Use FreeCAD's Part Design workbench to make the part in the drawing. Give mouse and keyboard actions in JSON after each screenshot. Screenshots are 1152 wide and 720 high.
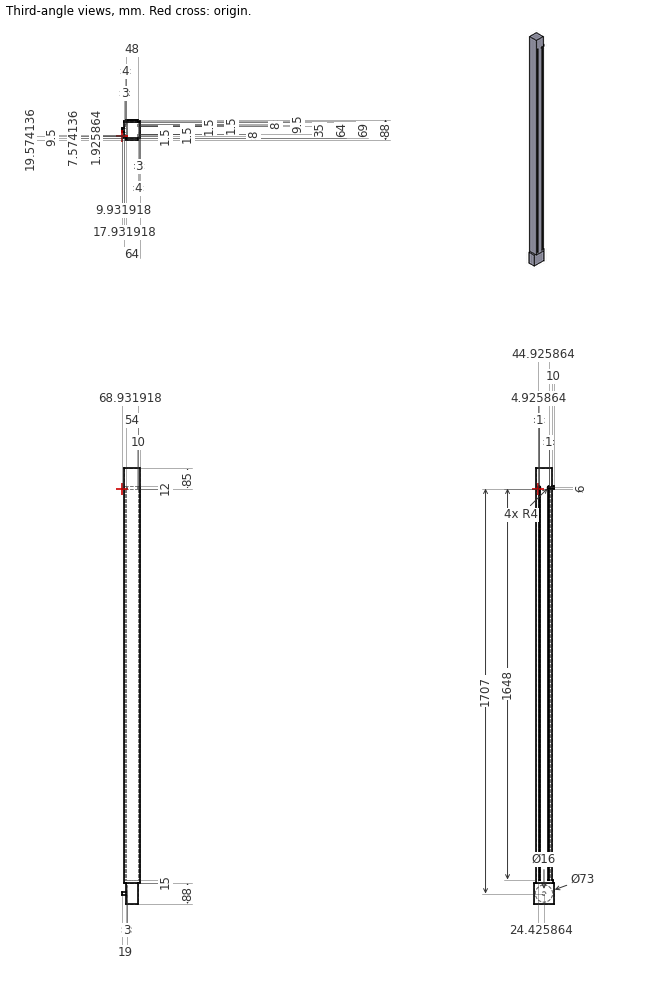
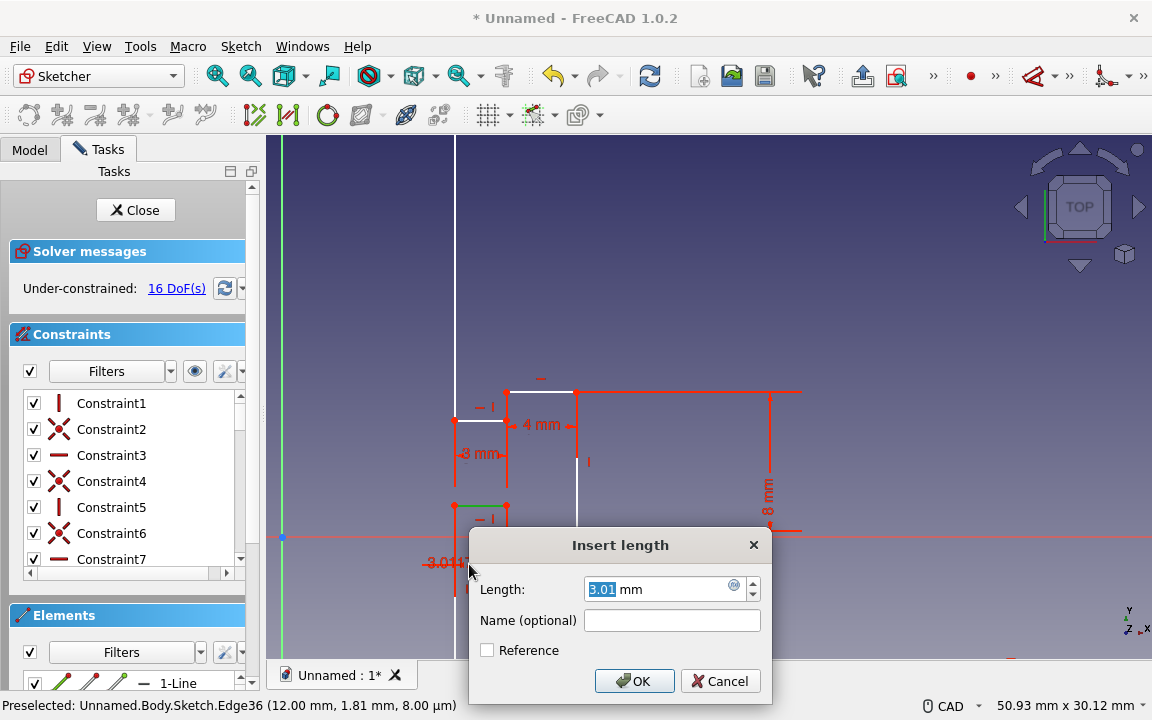
{"action": "type", "text": "3"}
{"action": "key", "text": "Return"}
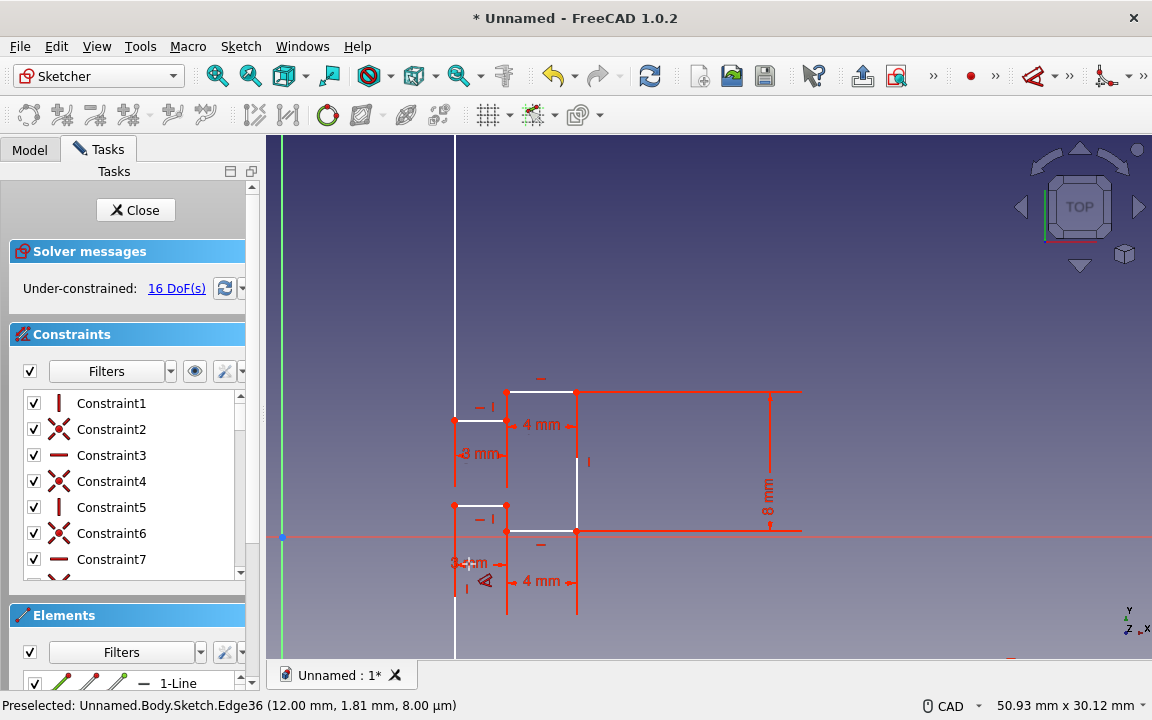
{"action": "scroll", "coordinate": [518, 520], "scroll_direction": "down", "scroll_amount": 6}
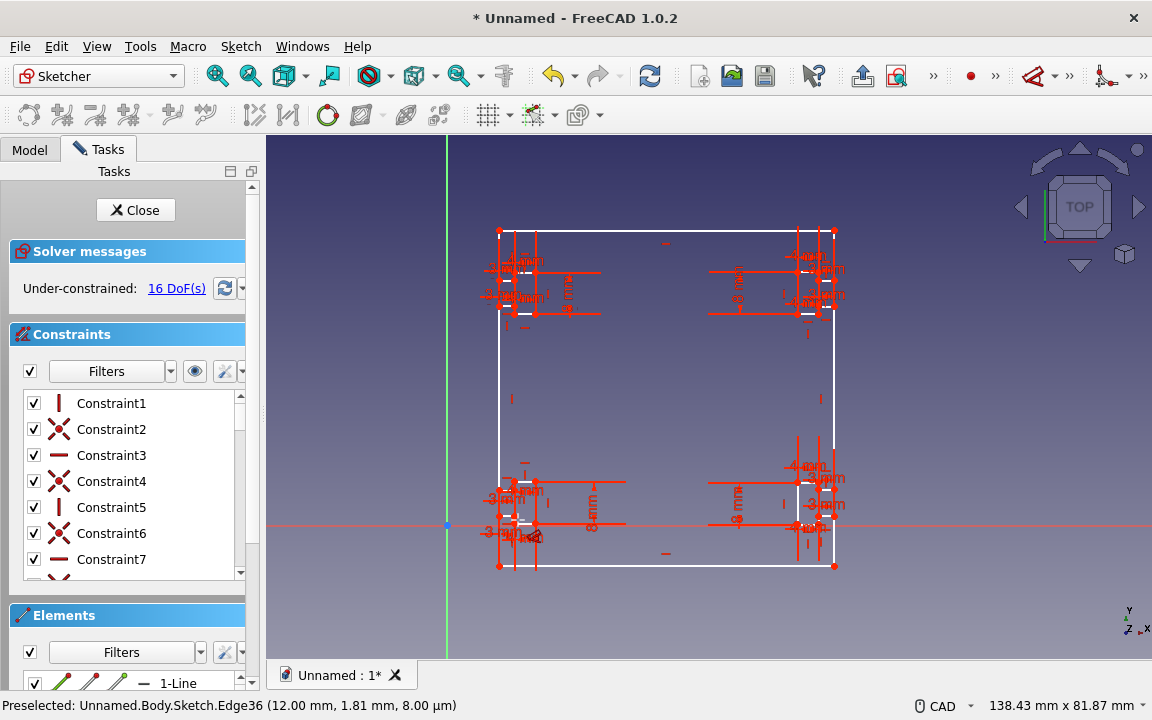
{"action": "left_click", "coordinate": [600, 566]}
{"action": "left_click", "coordinate": [667, 600]}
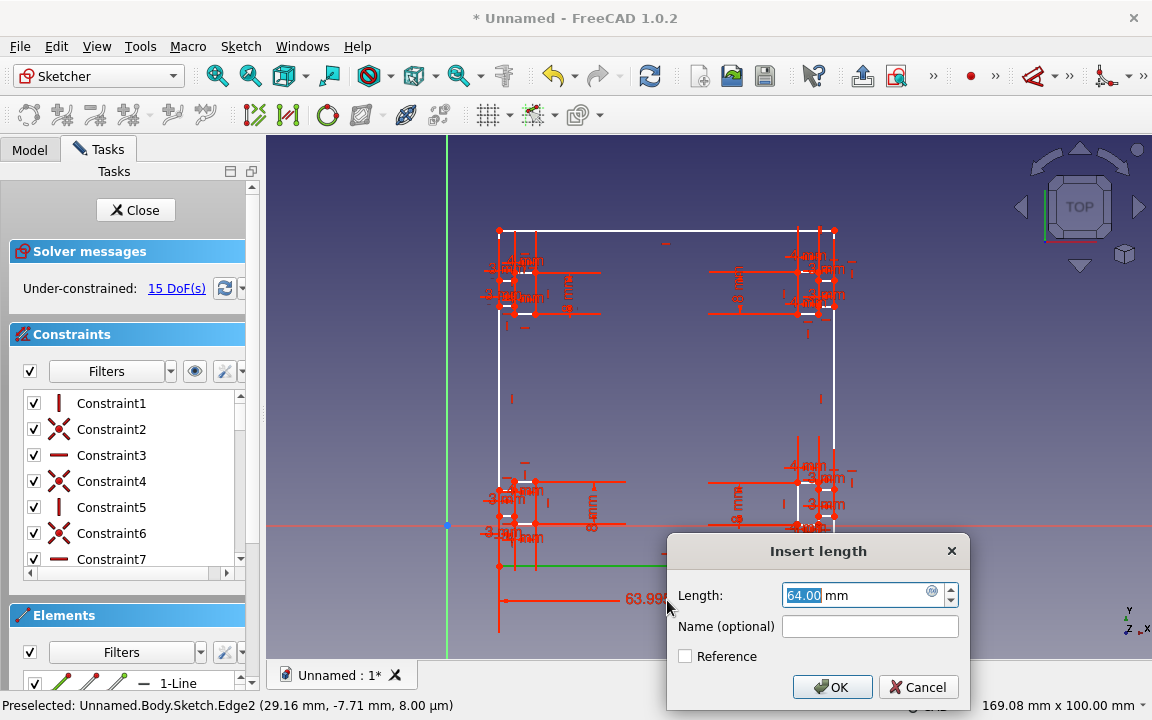
{"action": "type", "text": "64"}
{"action": "key", "text": "Return"}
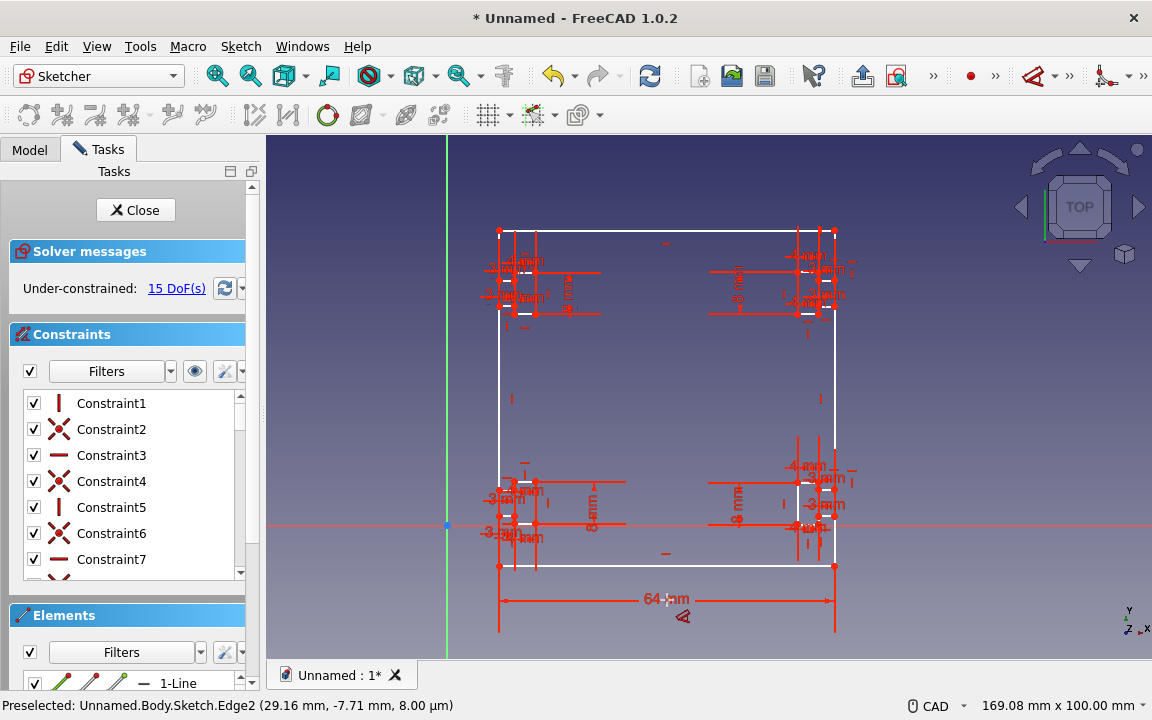
{"action": "left_click", "coordinate": [835, 435]}
{"action": "left_click", "coordinate": [869, 398]}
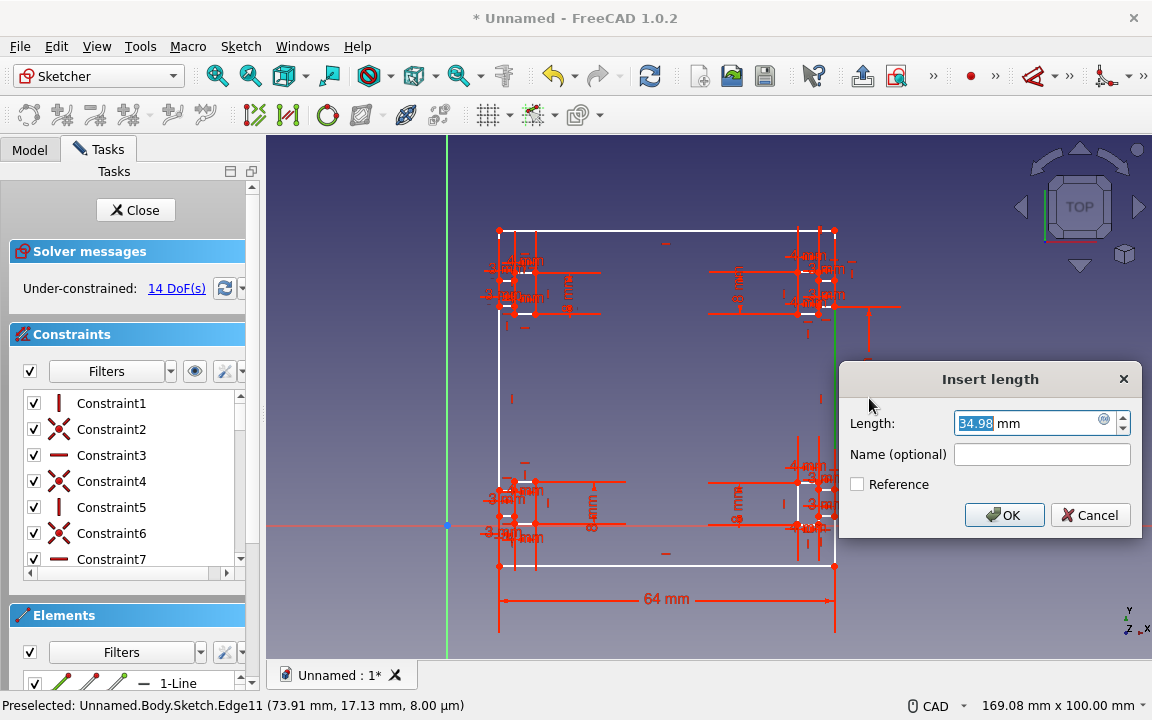
{"action": "type", "text": "35"}
{"action": "key", "text": "Return"}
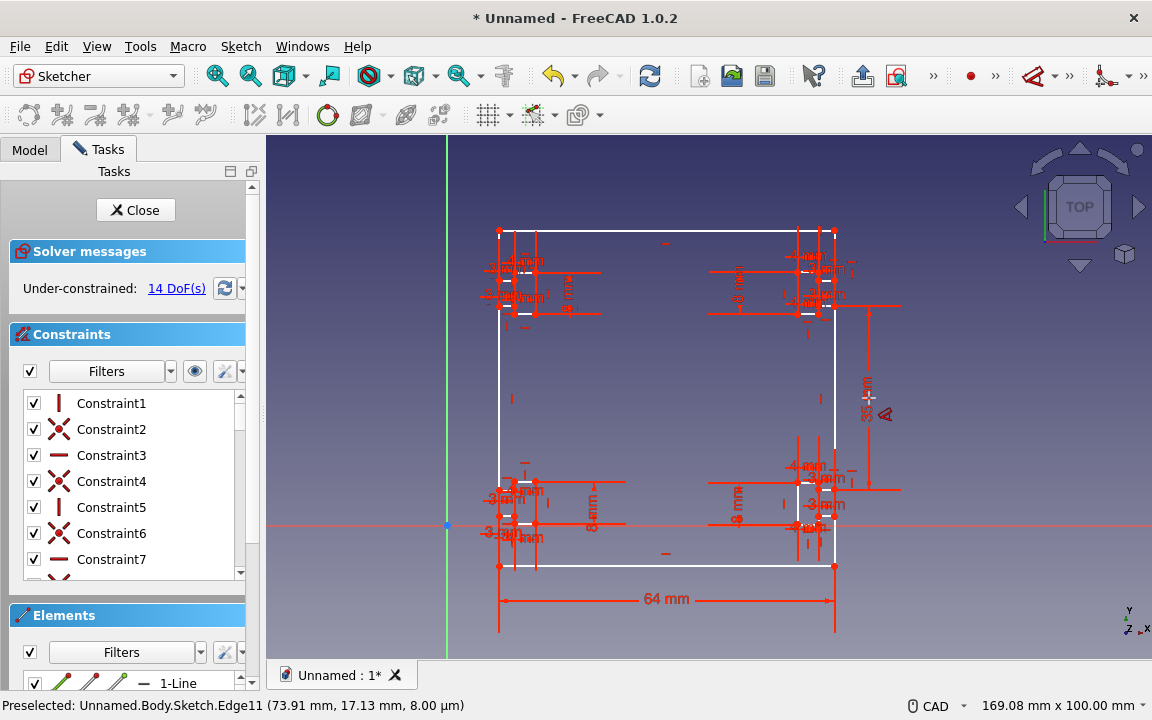
{"action": "left_click", "coordinate": [499, 362]}
{"action": "left_click", "coordinate": [465, 398]}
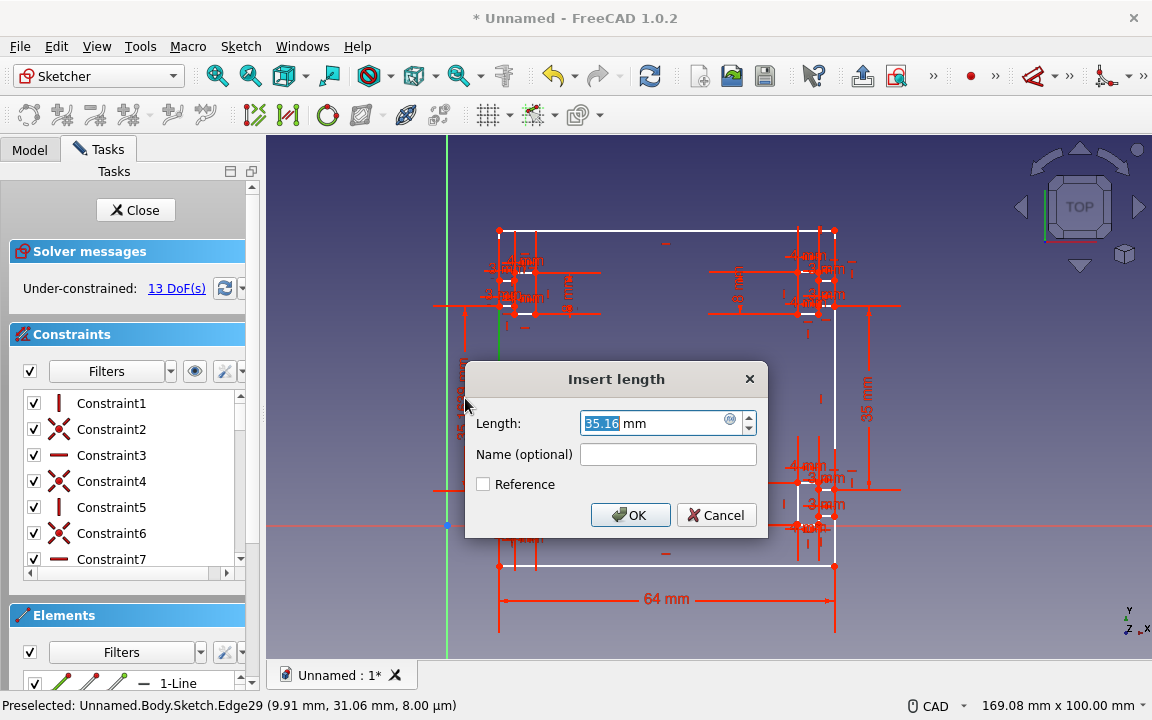
{"action": "type", "text": "35"}
{"action": "key", "text": "Return"}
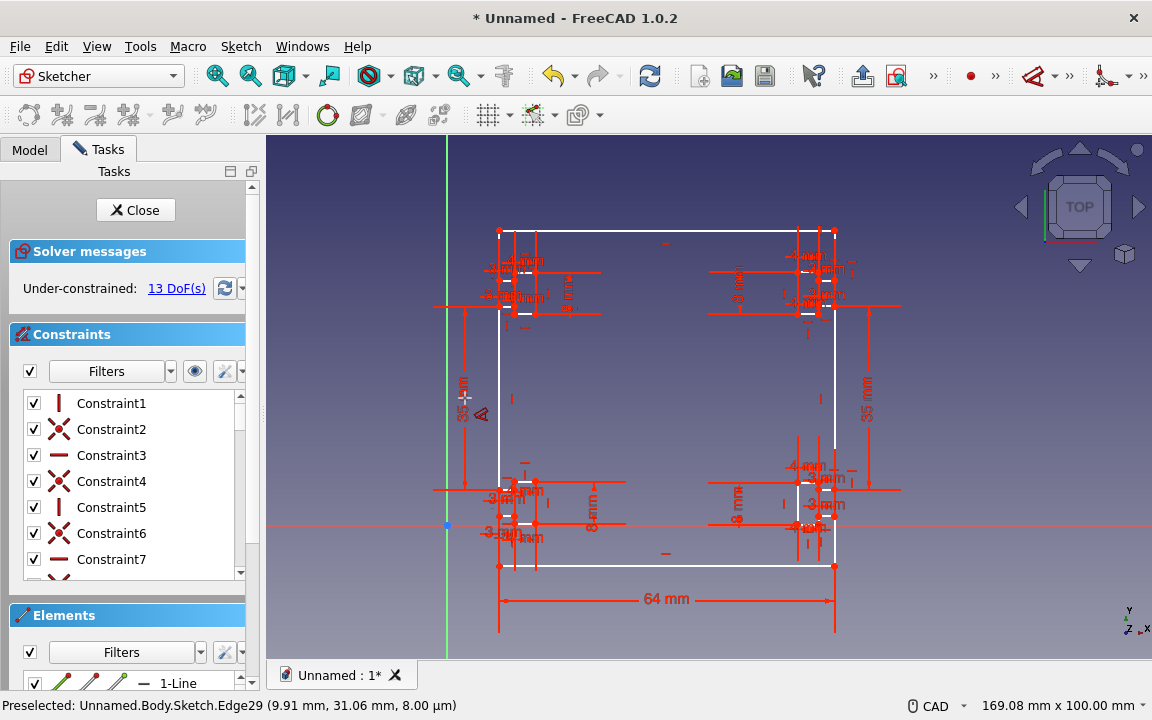
{"action": "left_click", "coordinate": [499, 551]}
{"action": "left_click", "coordinate": [417, 541]}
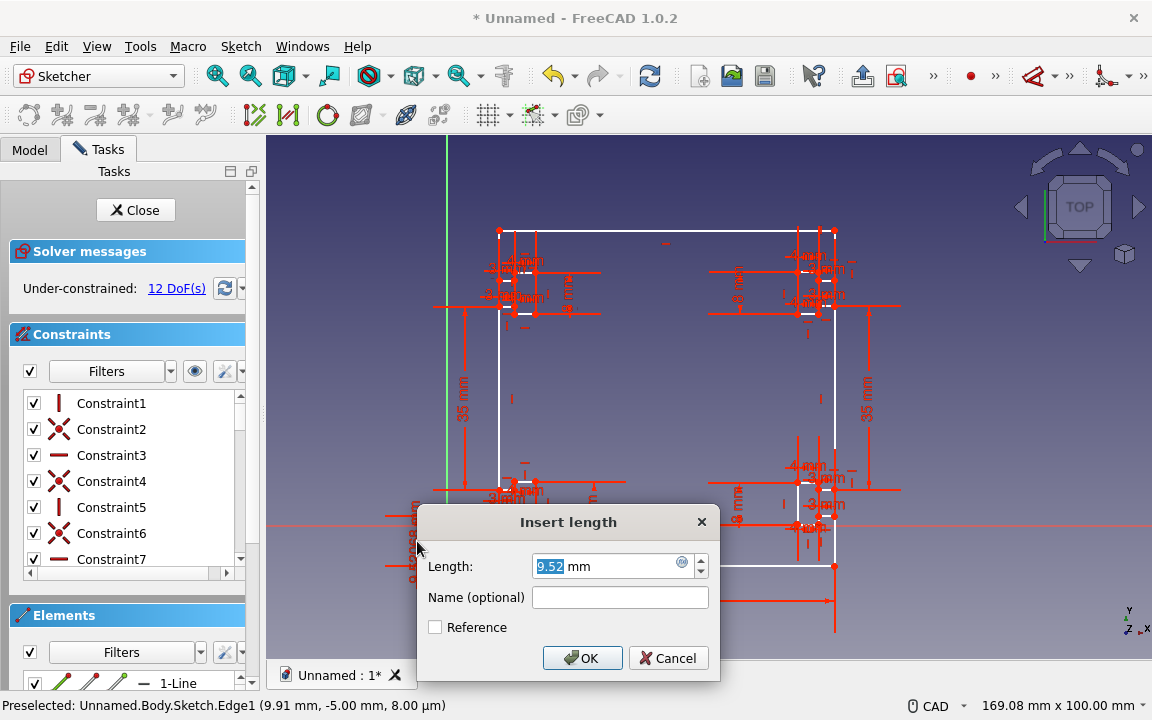
{"action": "type", "text": "9.5"}
{"action": "key", "text": "Return"}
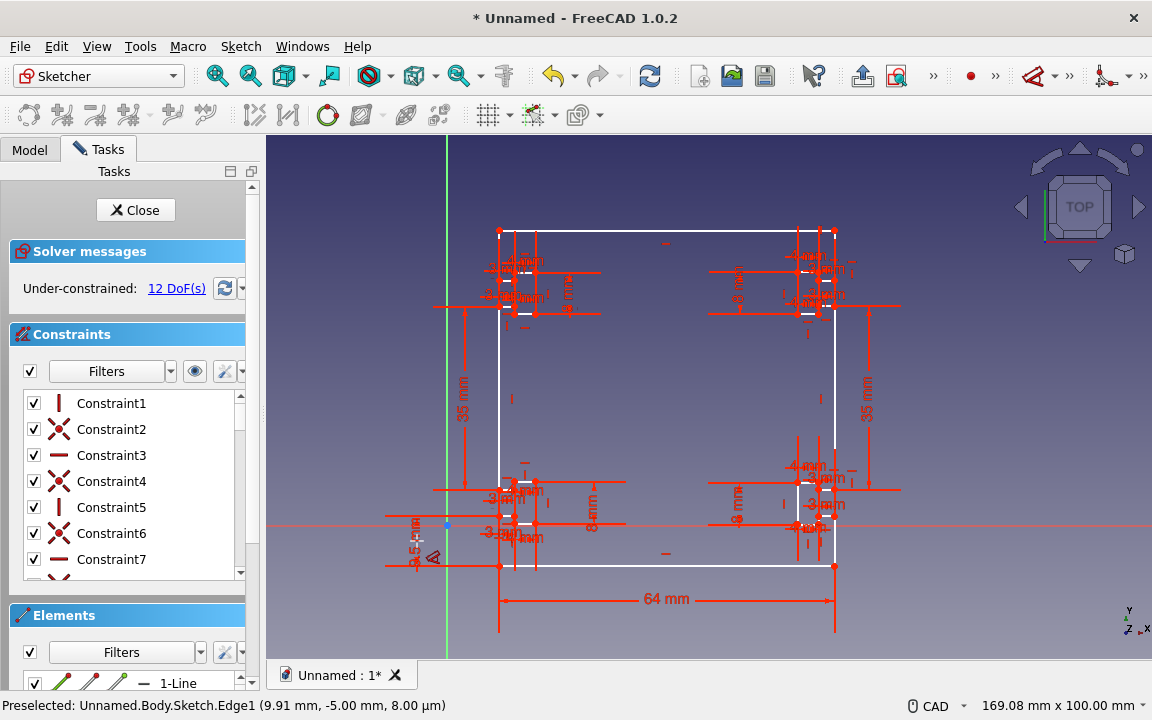
{"action": "left_click", "coordinate": [835, 551]}
{"action": "left_click", "coordinate": [869, 553]}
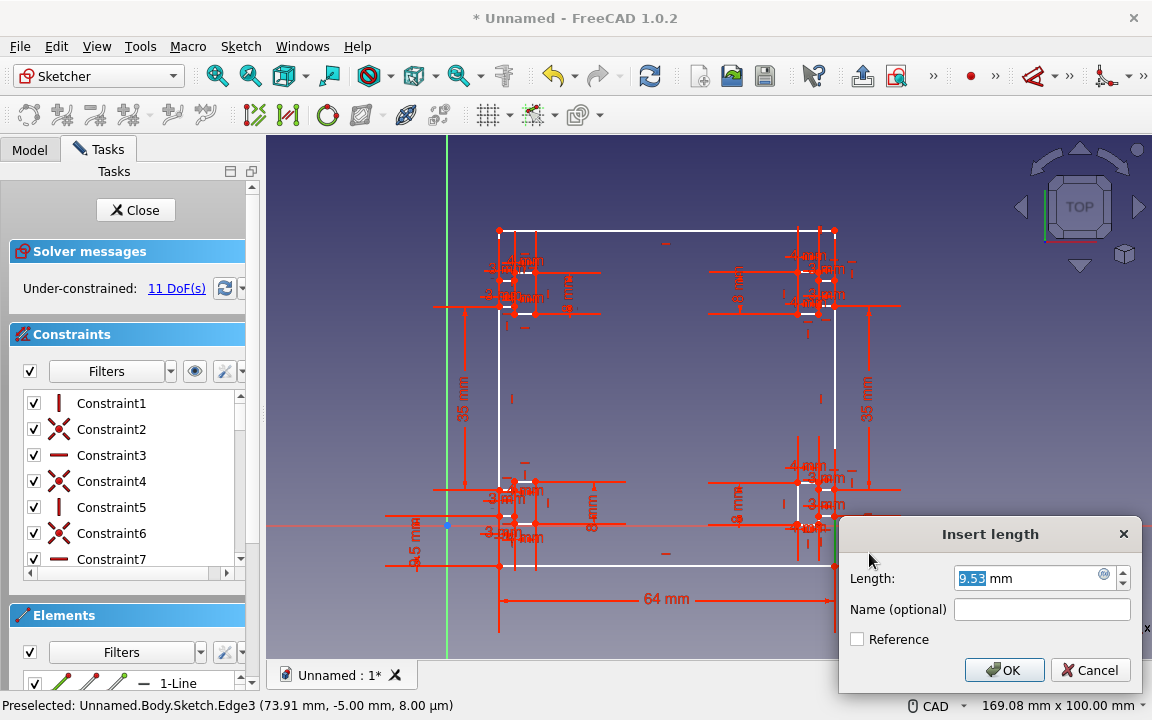
{"action": "type", "text": "9.5"}
{"action": "key", "text": "Return"}